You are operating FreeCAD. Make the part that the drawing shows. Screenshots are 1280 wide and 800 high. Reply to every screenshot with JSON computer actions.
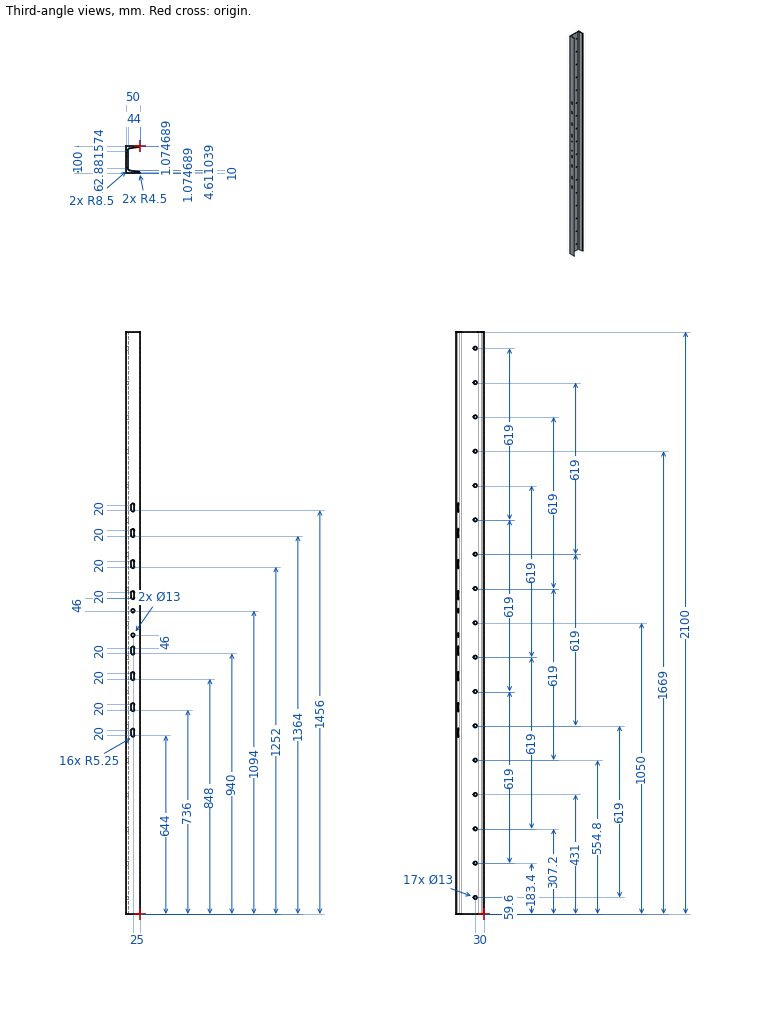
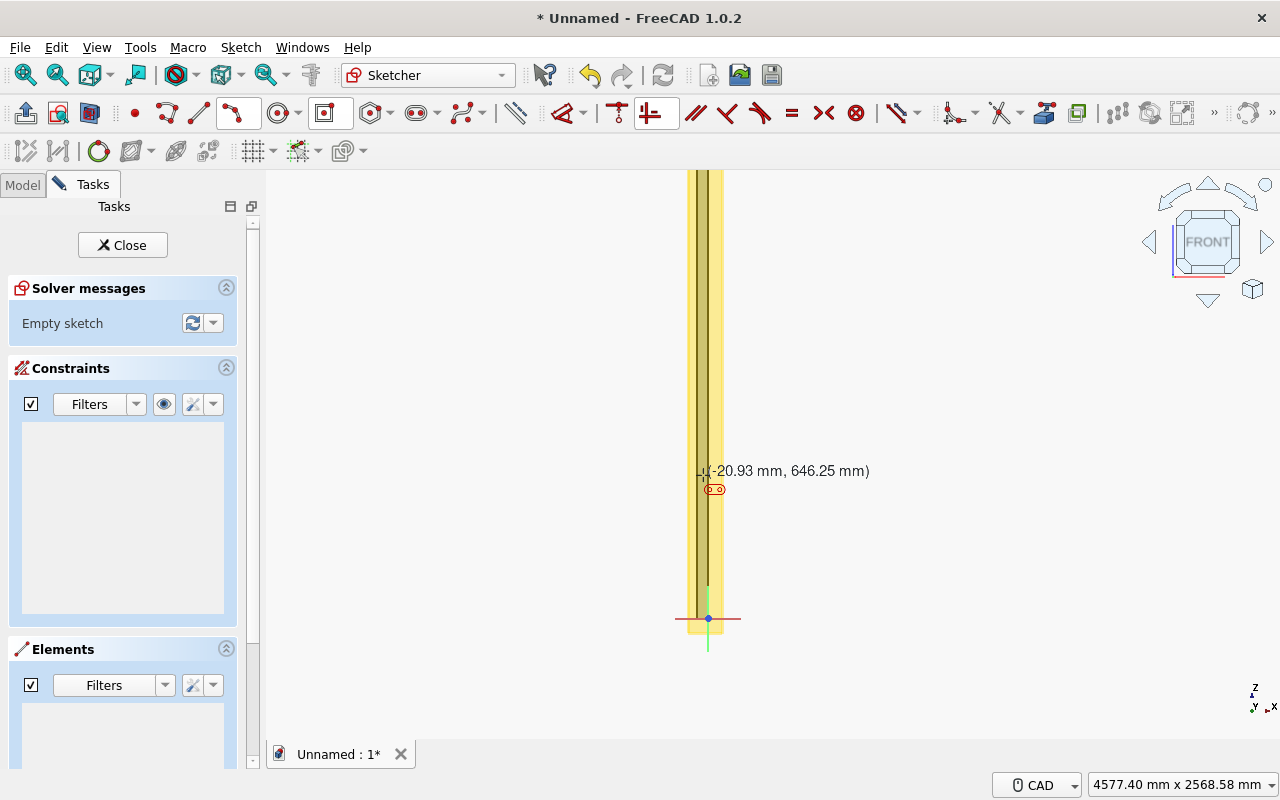
{"action": "scroll", "coordinate": [703, 476], "scroll_direction": "up", "scroll_amount": 6}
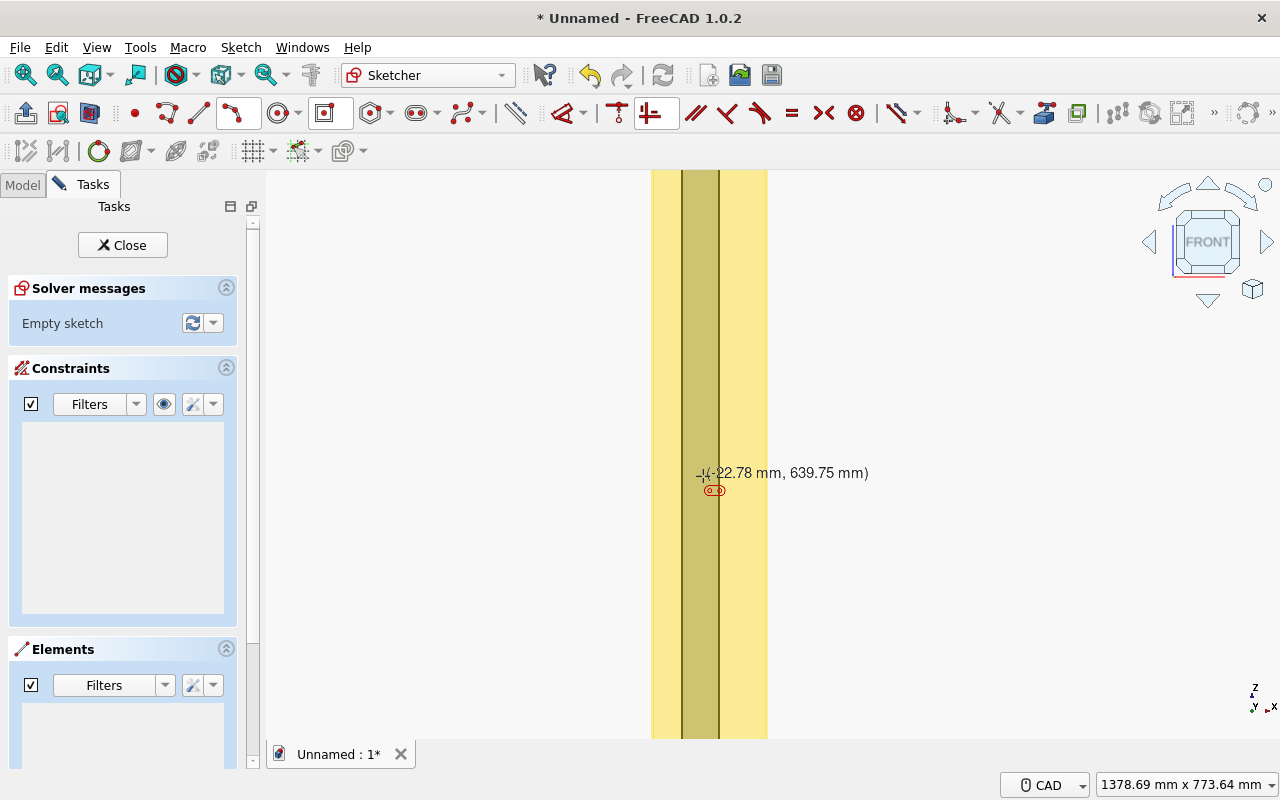
{"action": "left_click", "coordinate": [700, 475]}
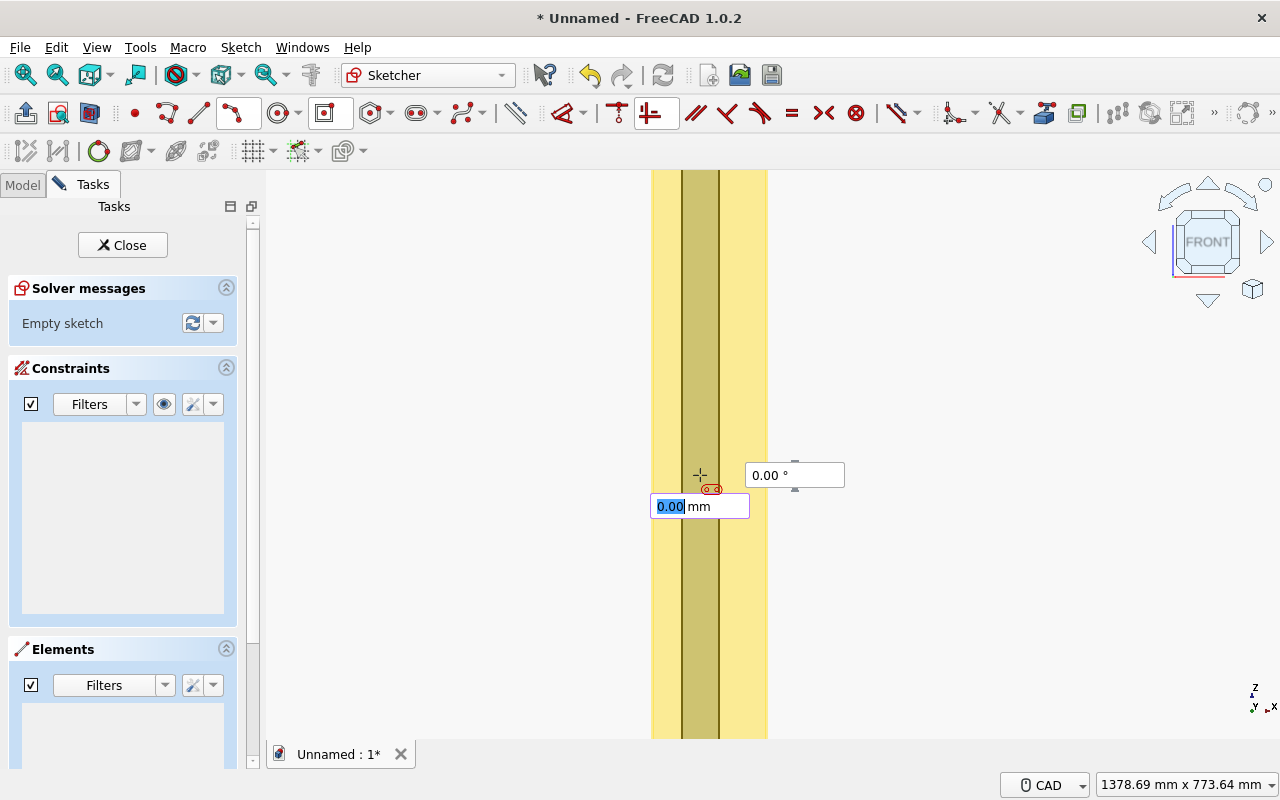
{"action": "left_click", "coordinate": [700, 460]}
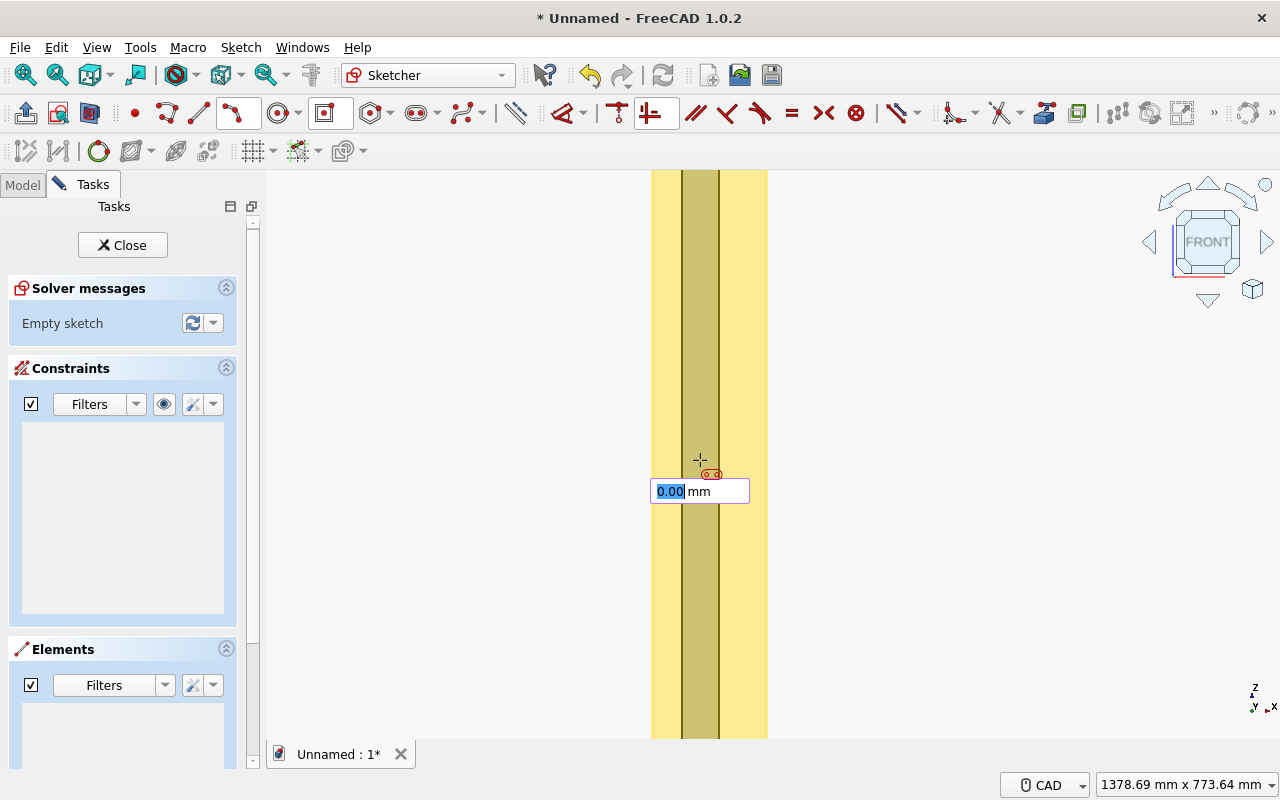
{"action": "scroll", "coordinate": [697, 468], "scroll_direction": "up", "scroll_amount": 8}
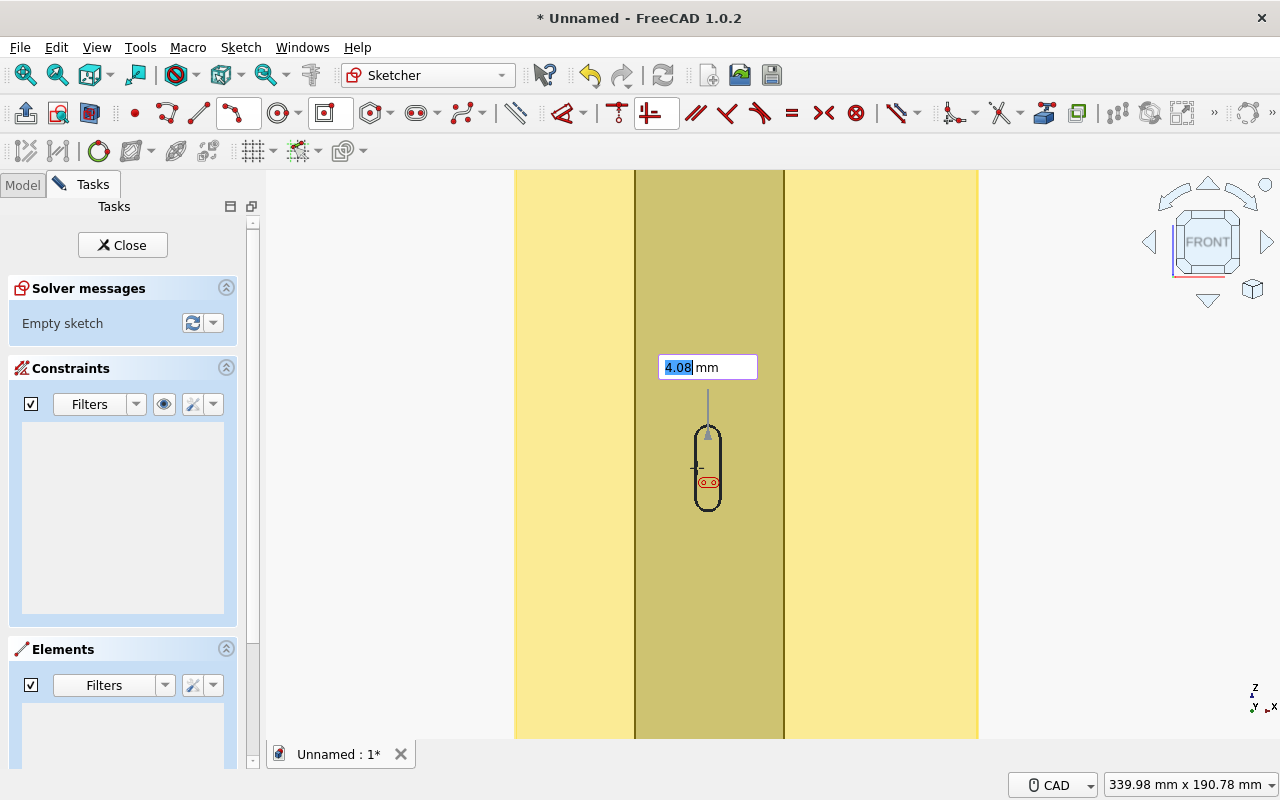
{"action": "left_click", "coordinate": [693, 464]}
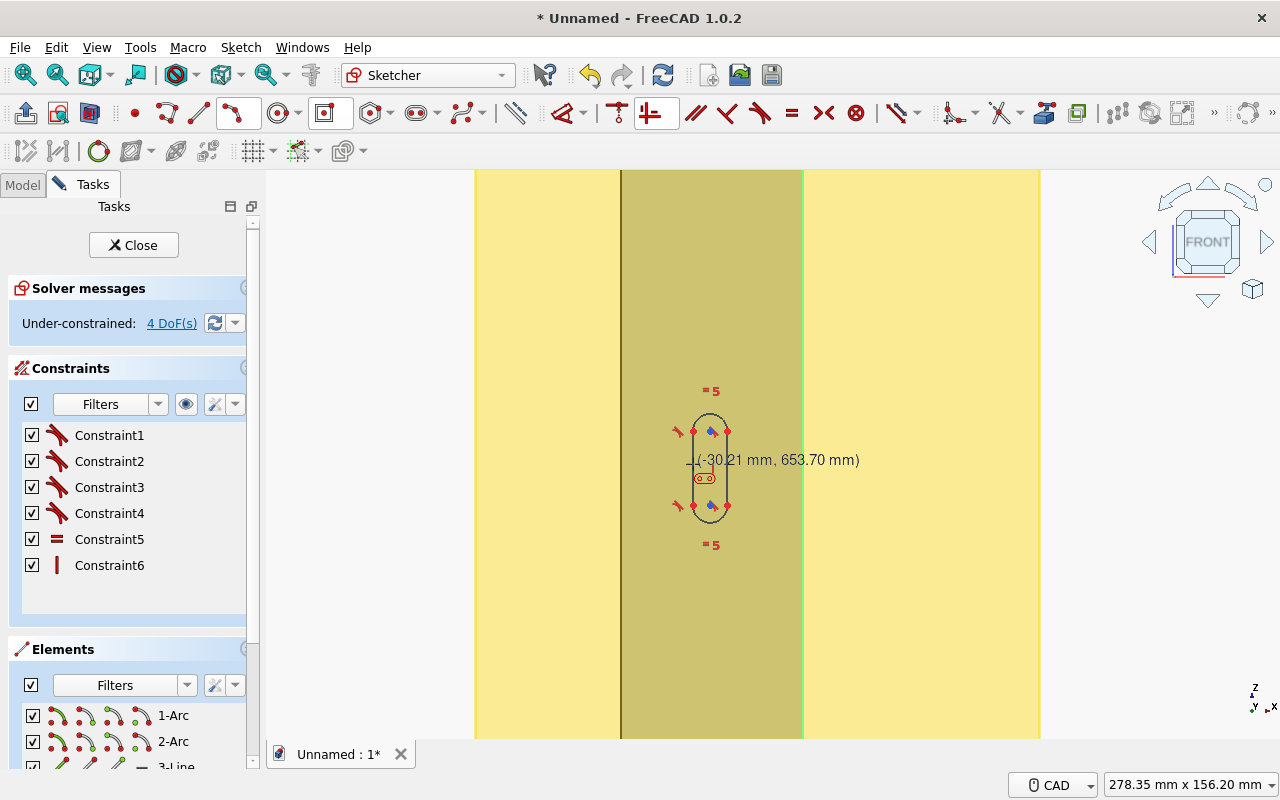
{"action": "scroll", "coordinate": [702, 474], "scroll_direction": "down", "scroll_amount": 14}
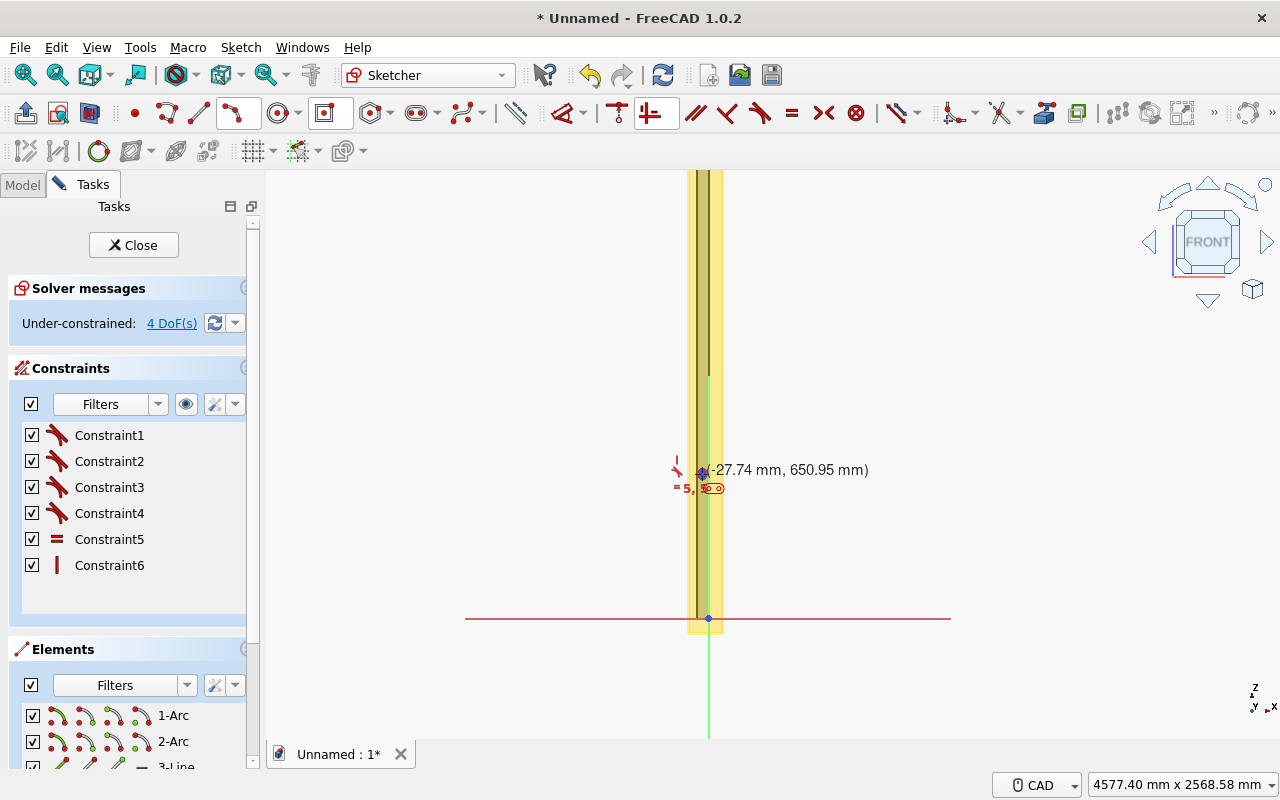
{"action": "scroll", "coordinate": [703, 456], "scroll_direction": "up", "scroll_amount": 15}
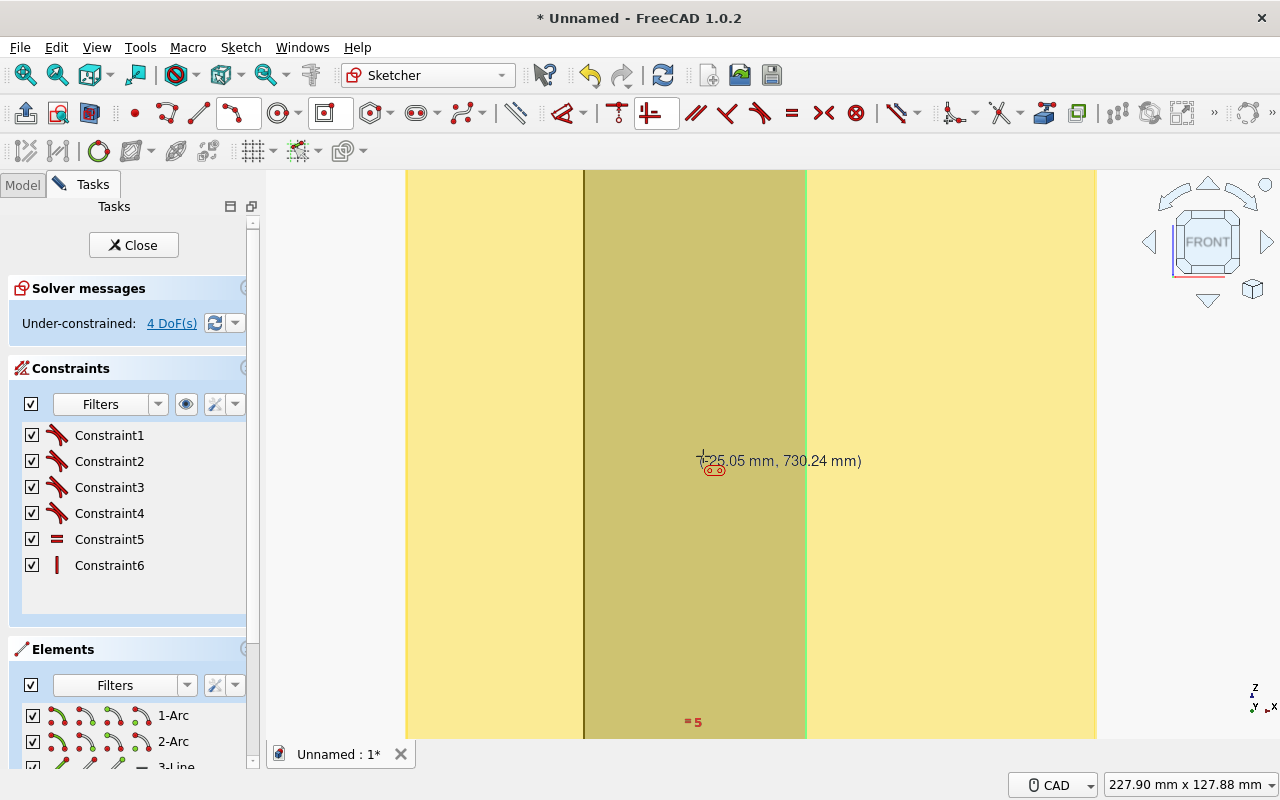
{"action": "scroll", "coordinate": [703, 456], "scroll_direction": "down", "scroll_amount": 15}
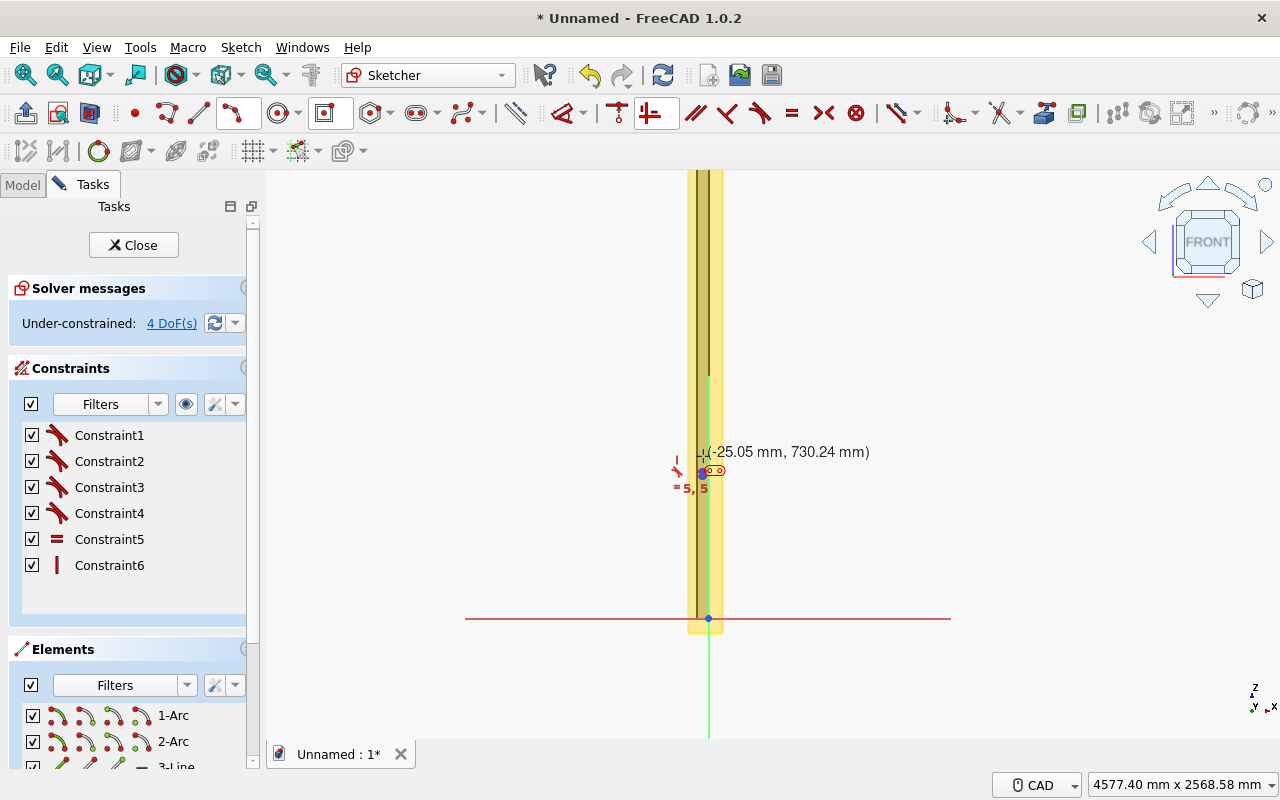
{"action": "scroll", "coordinate": [703, 456], "scroll_direction": "up", "scroll_amount": 6}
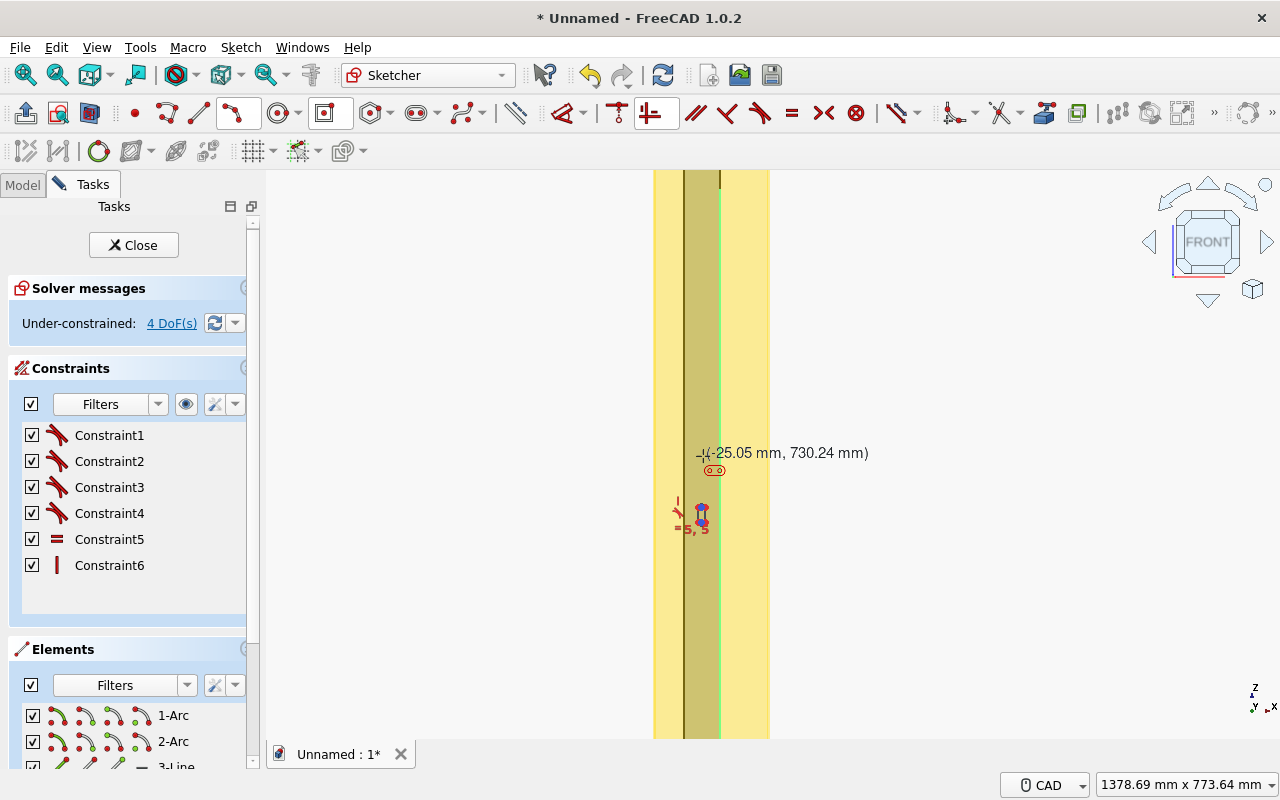
{"action": "left_click", "coordinate": [702, 454]}